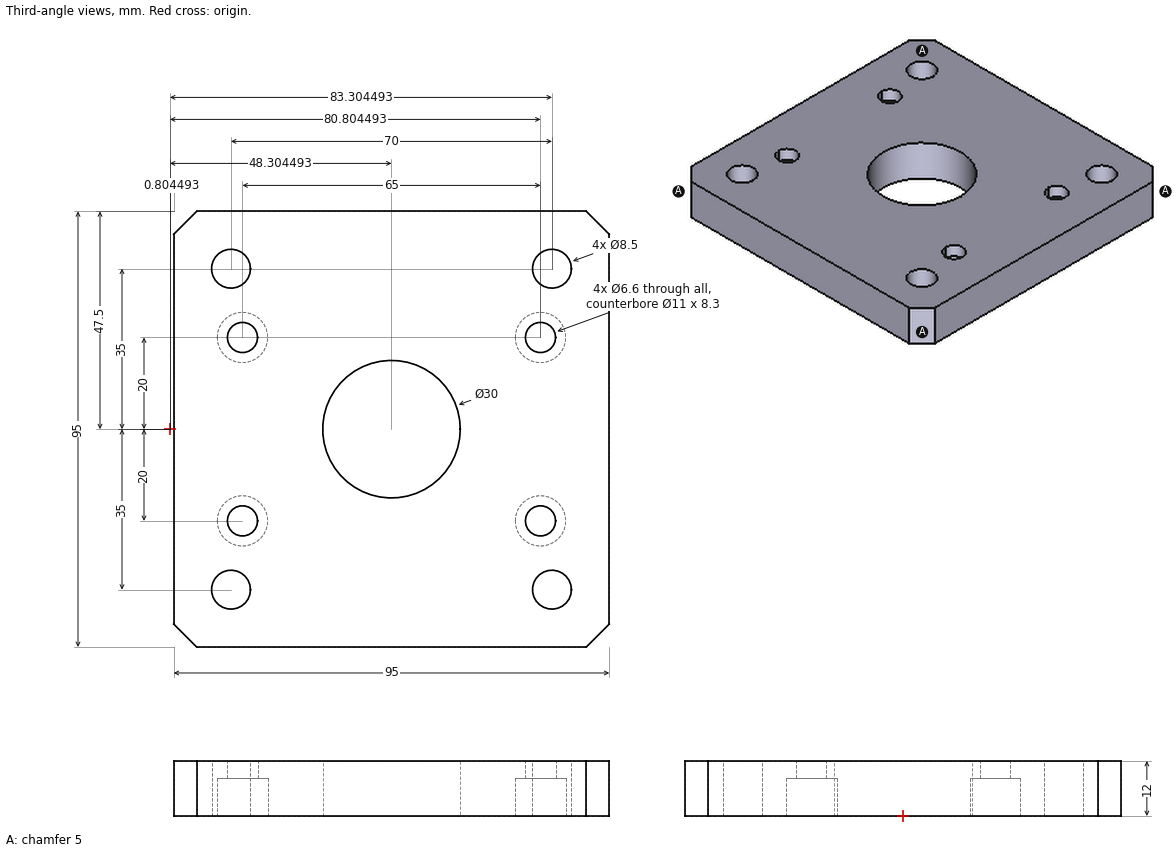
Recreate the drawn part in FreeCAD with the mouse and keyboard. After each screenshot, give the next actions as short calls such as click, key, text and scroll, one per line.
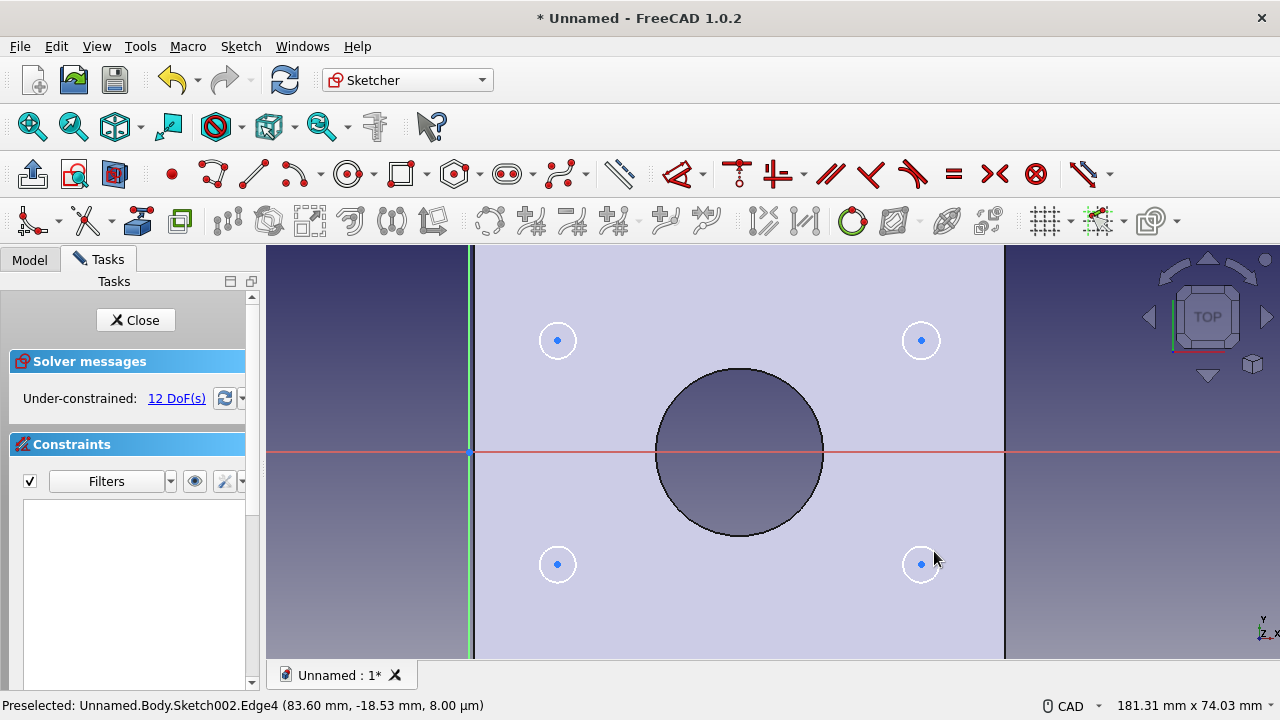
click(934, 328)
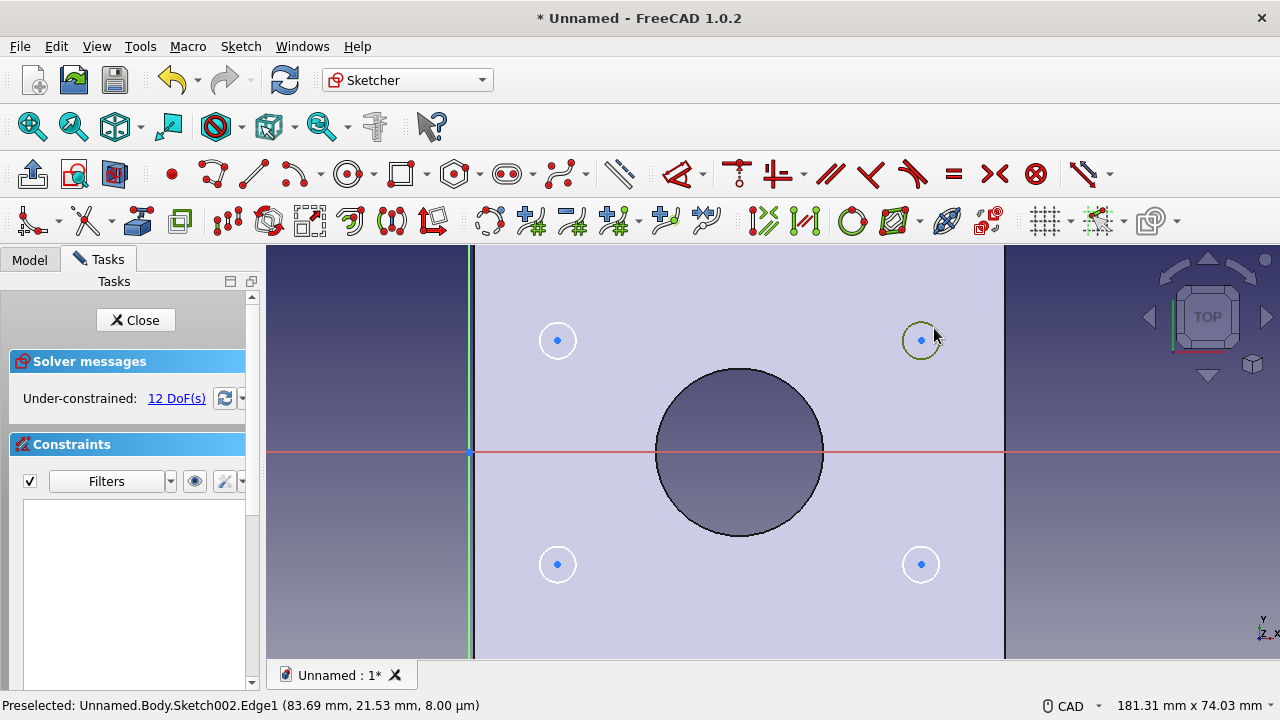
click(571, 328)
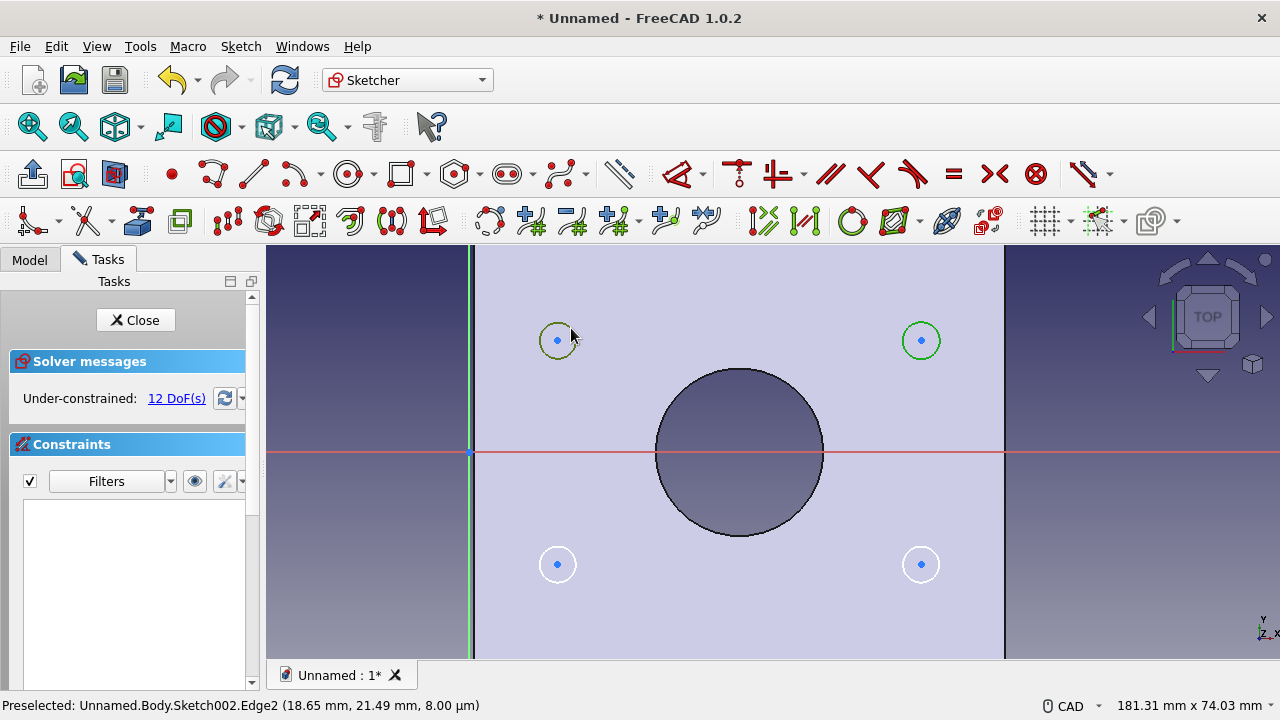
click(570, 552)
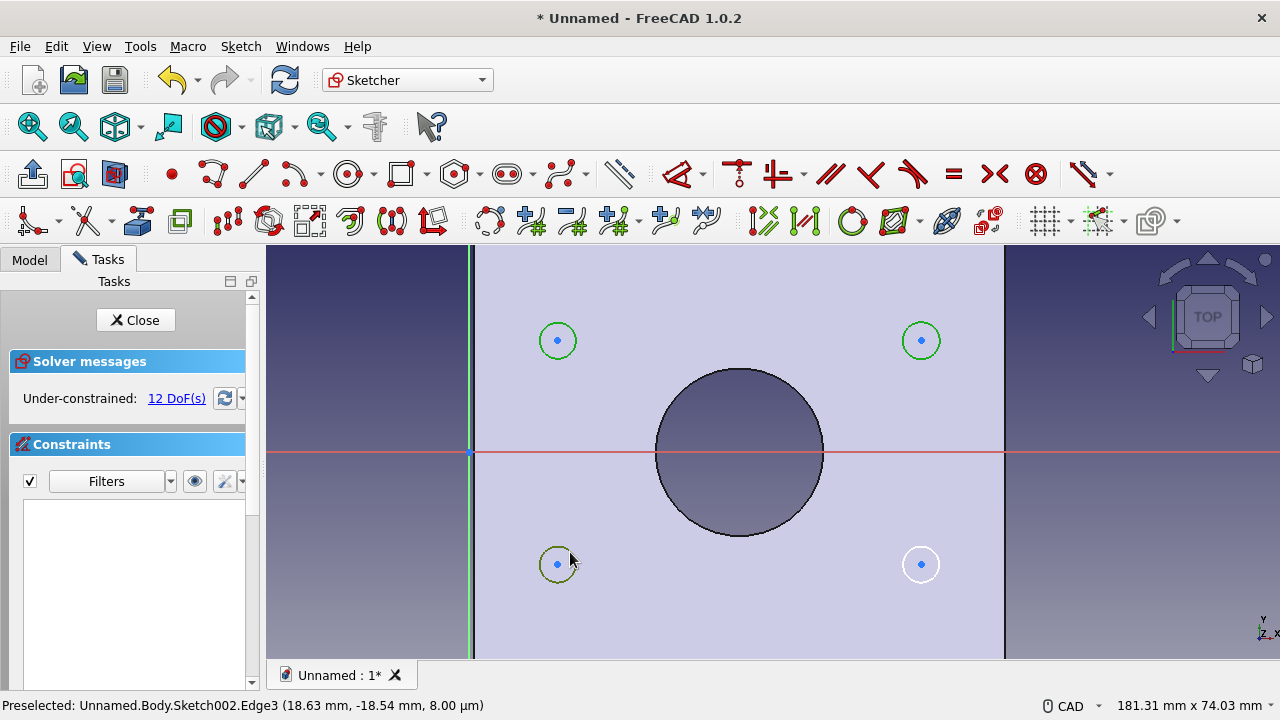
click(934, 552)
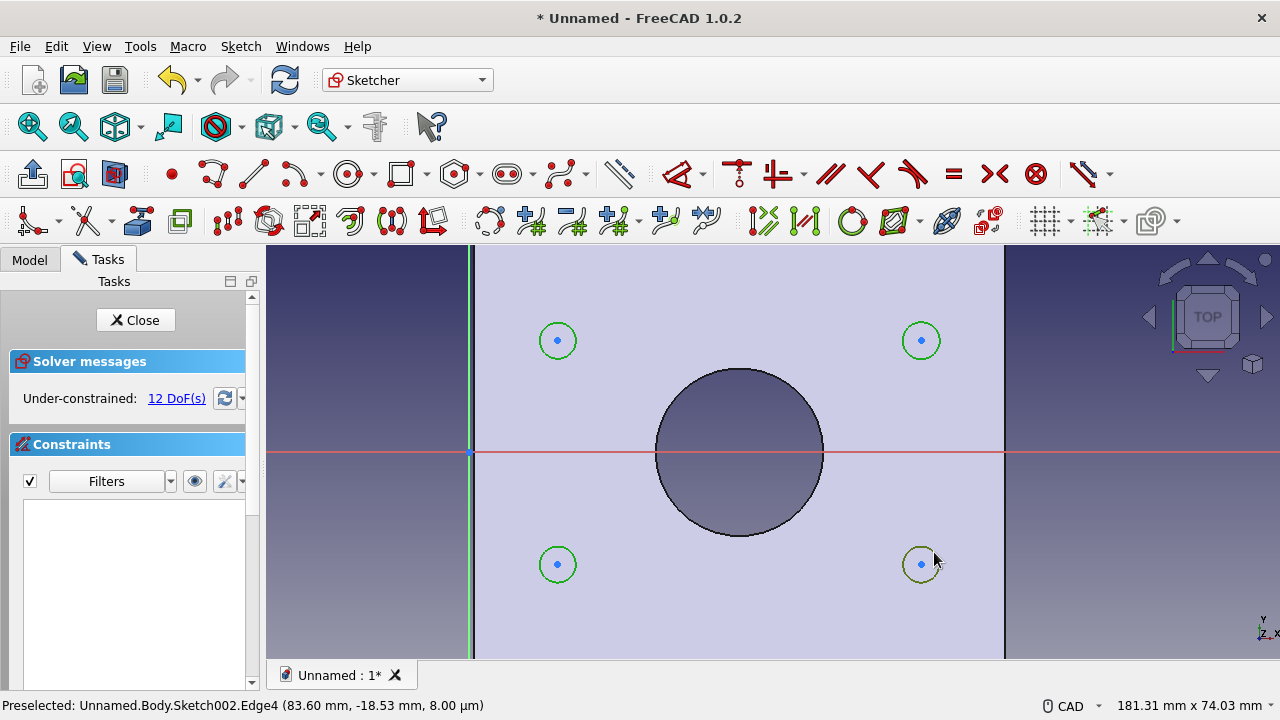
key(e)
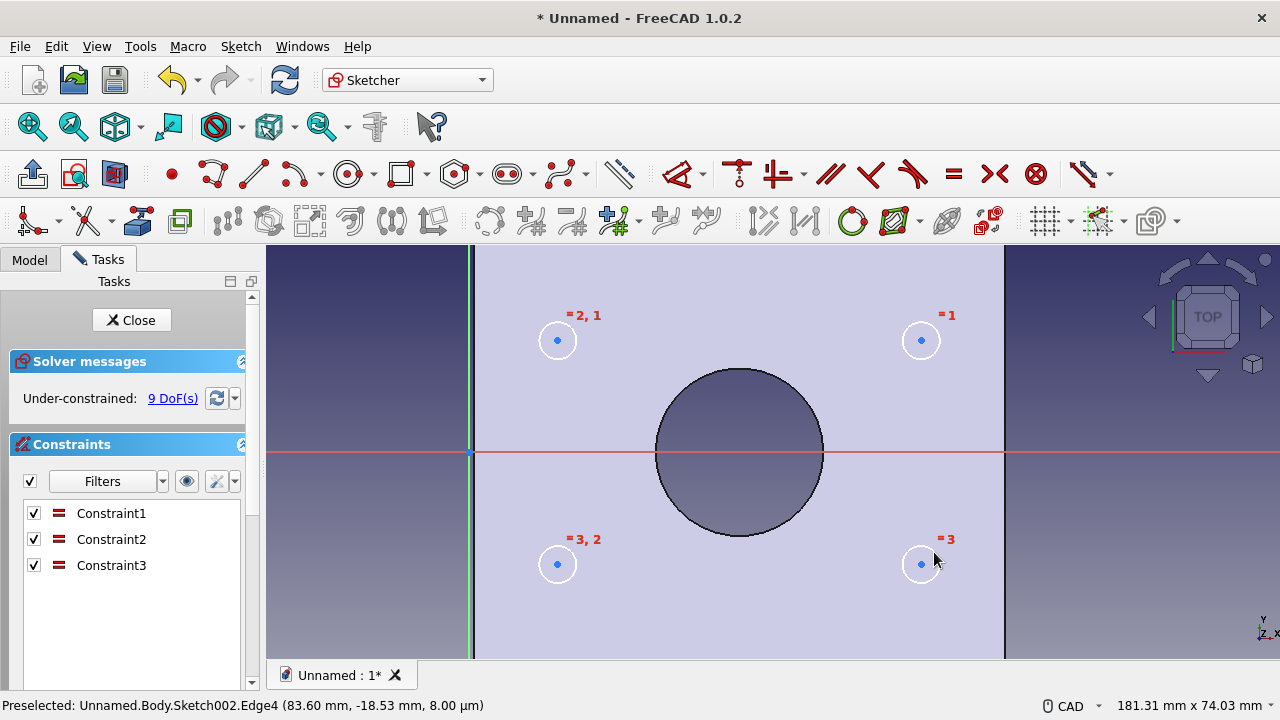
click(921, 341)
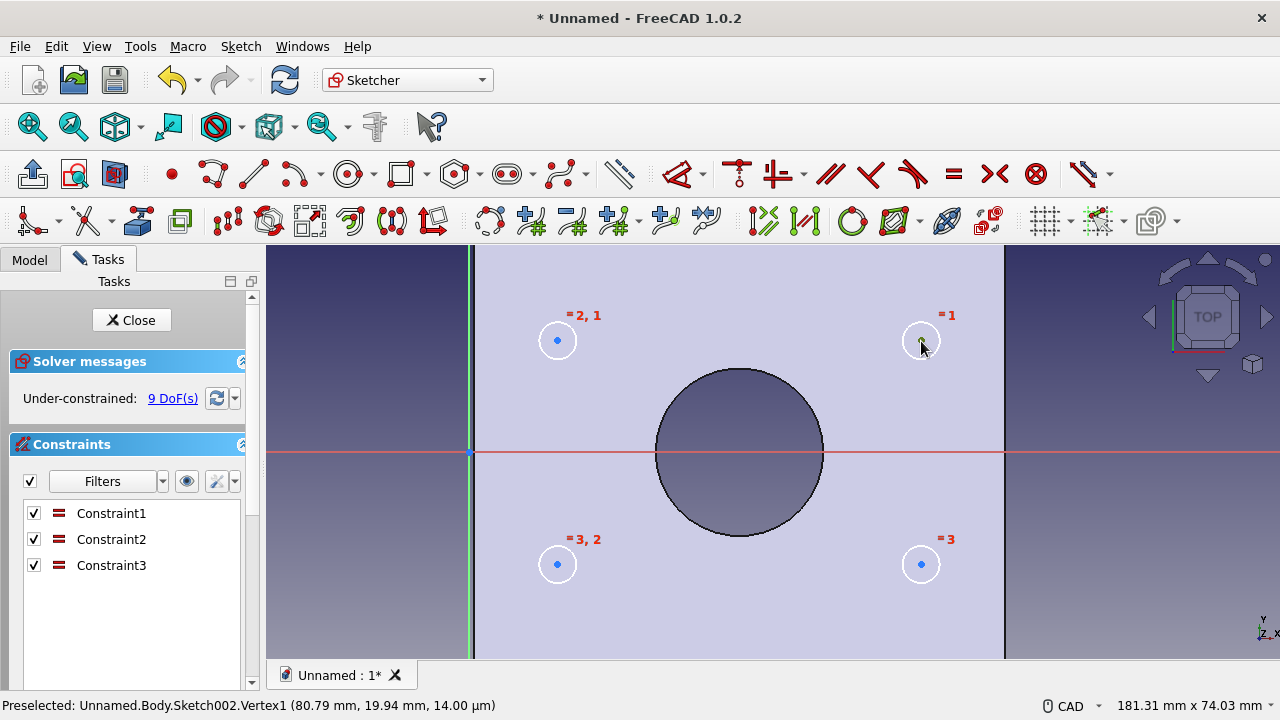
click(558, 341)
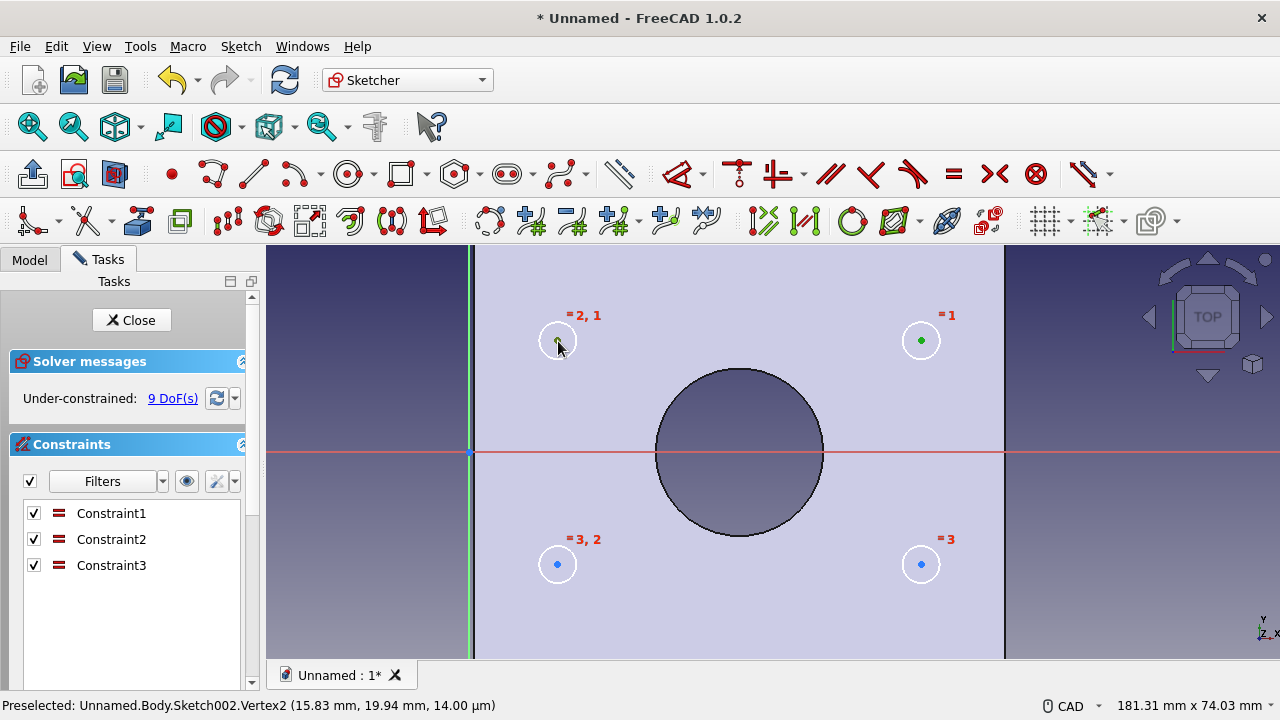
key(h)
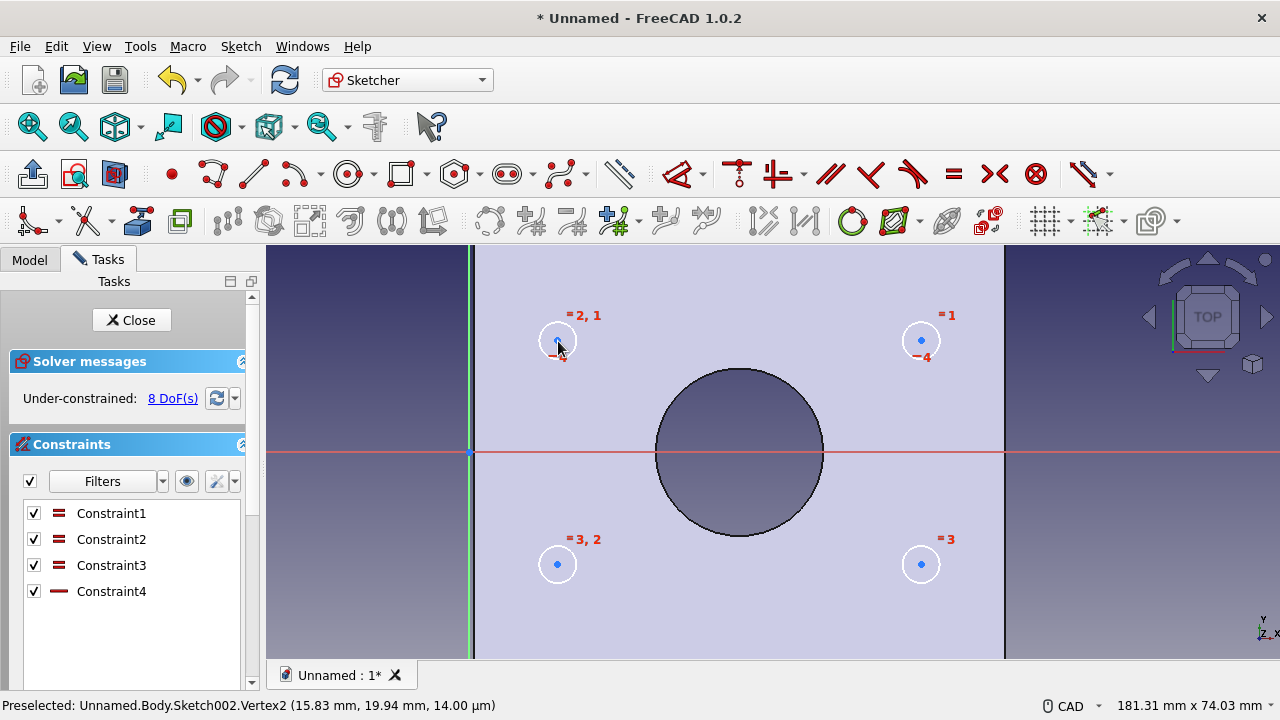
click(558, 341)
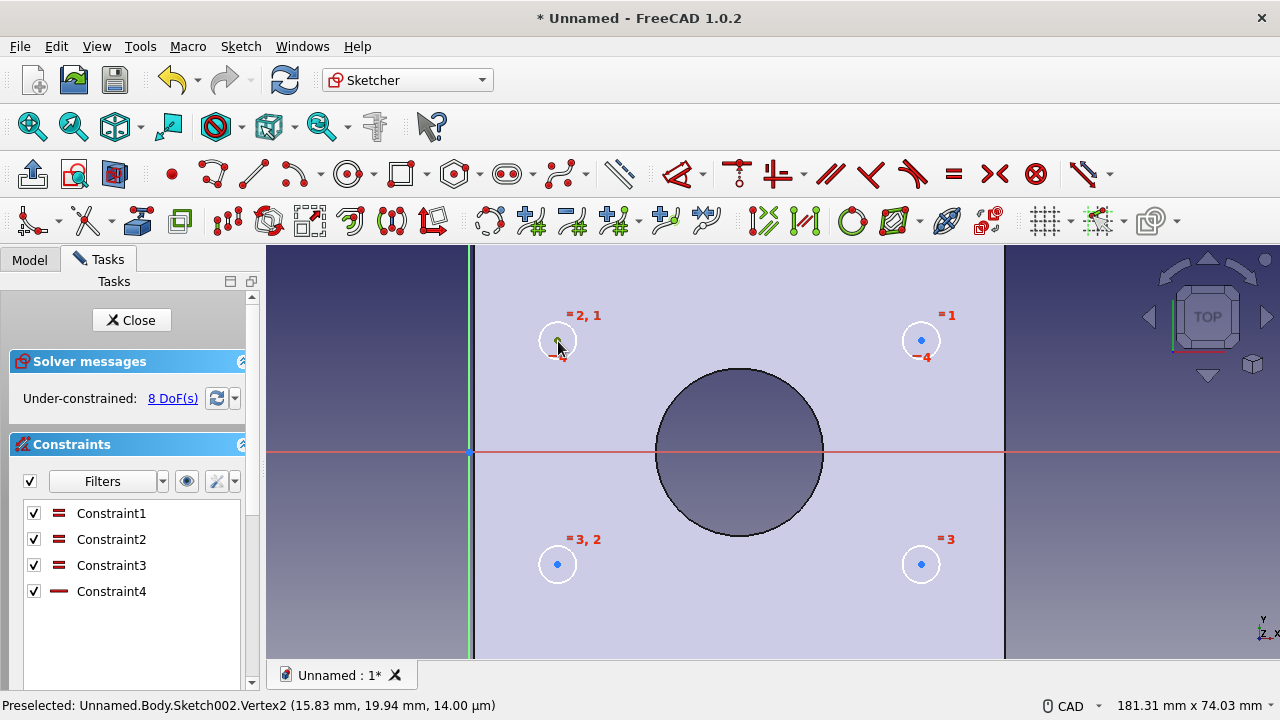
click(558, 565)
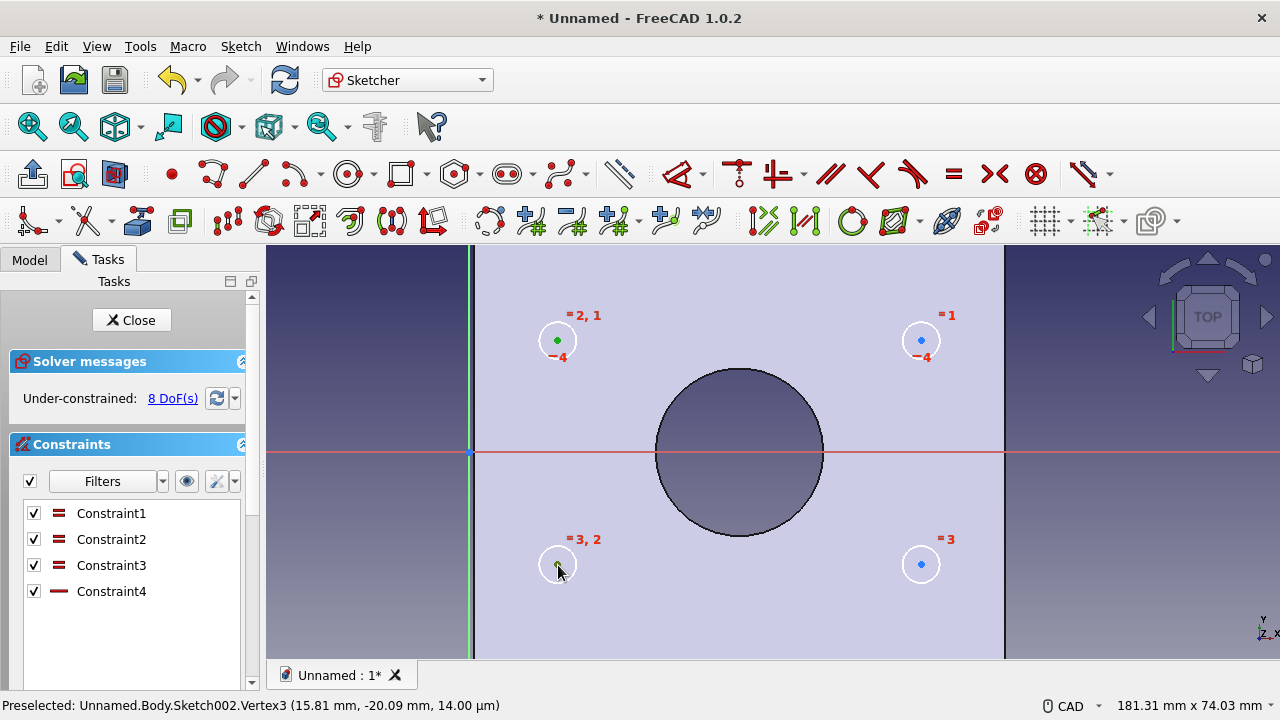
key(v)